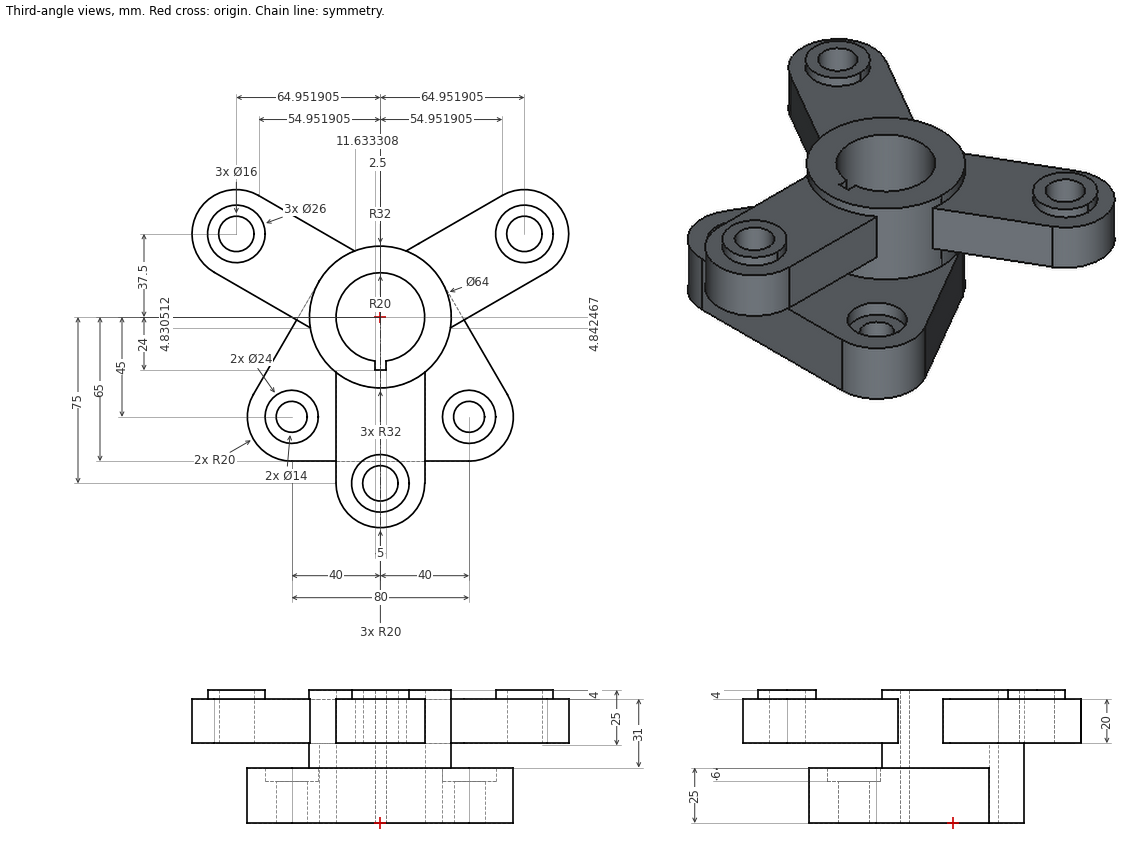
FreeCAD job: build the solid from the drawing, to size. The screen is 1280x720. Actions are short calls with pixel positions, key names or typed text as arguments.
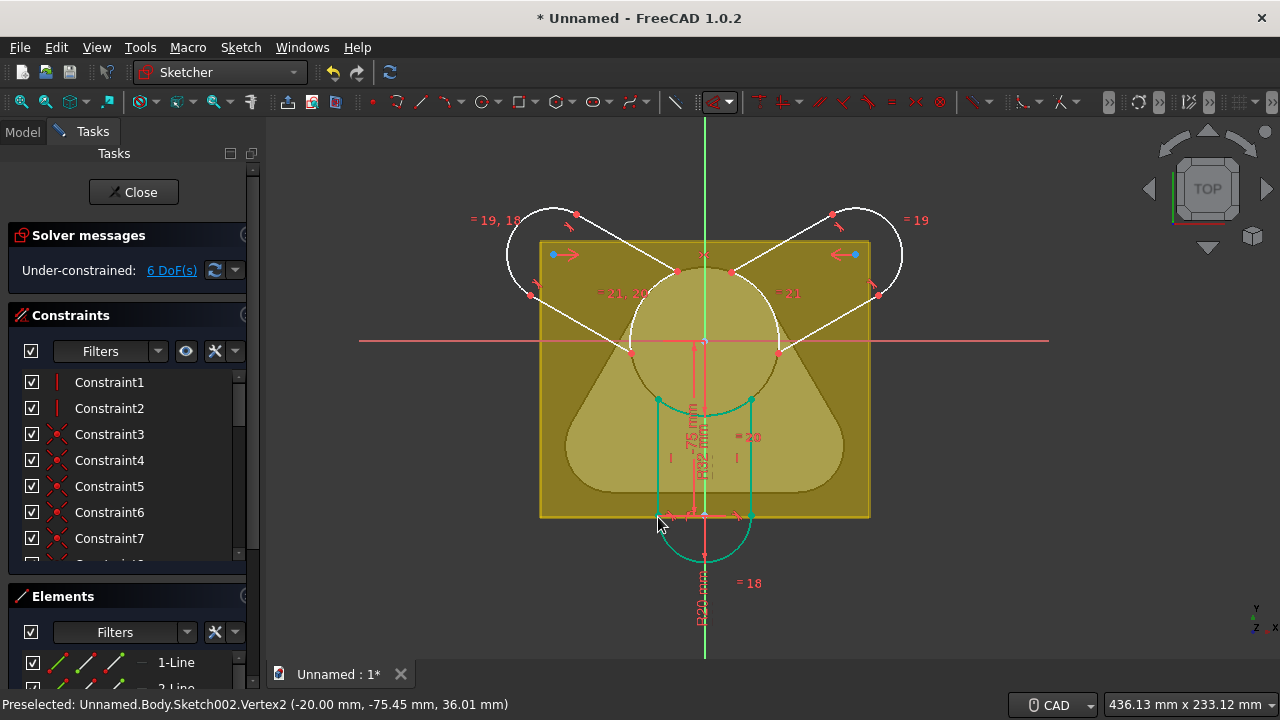
click(554, 255)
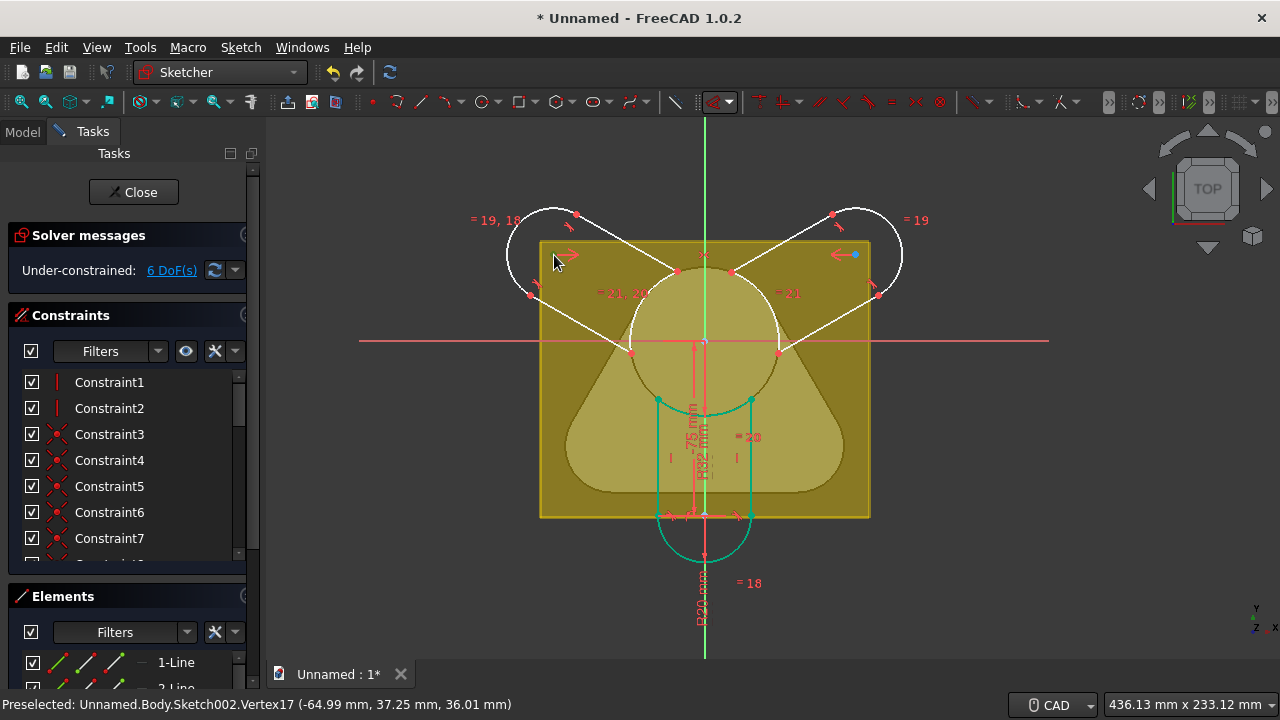
key(i)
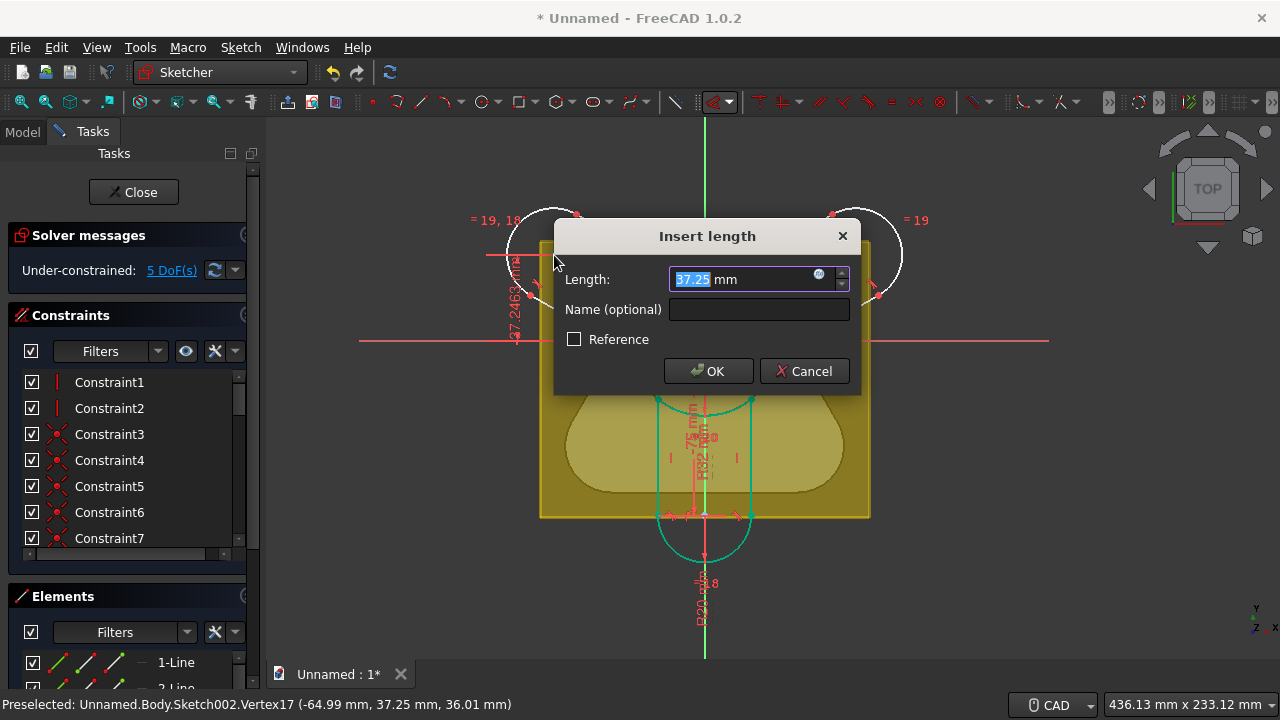
text(37.5)
key(Return)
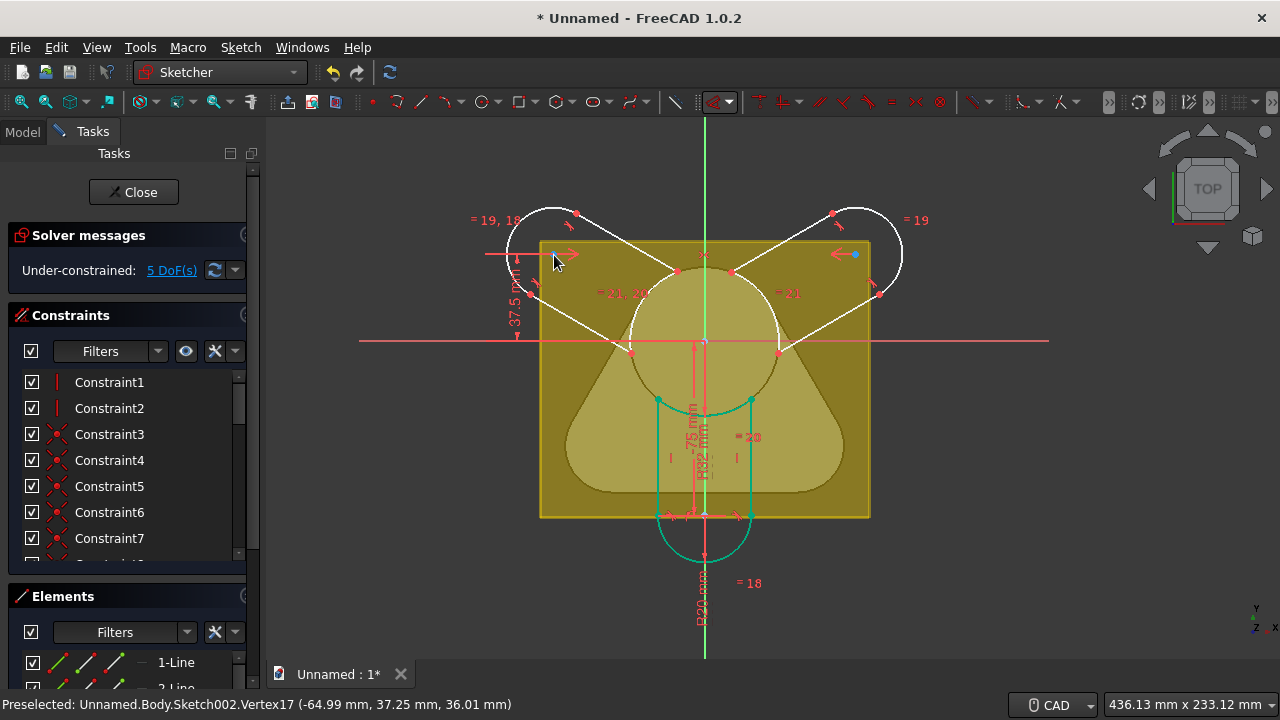
scroll(631, 353, up, 7)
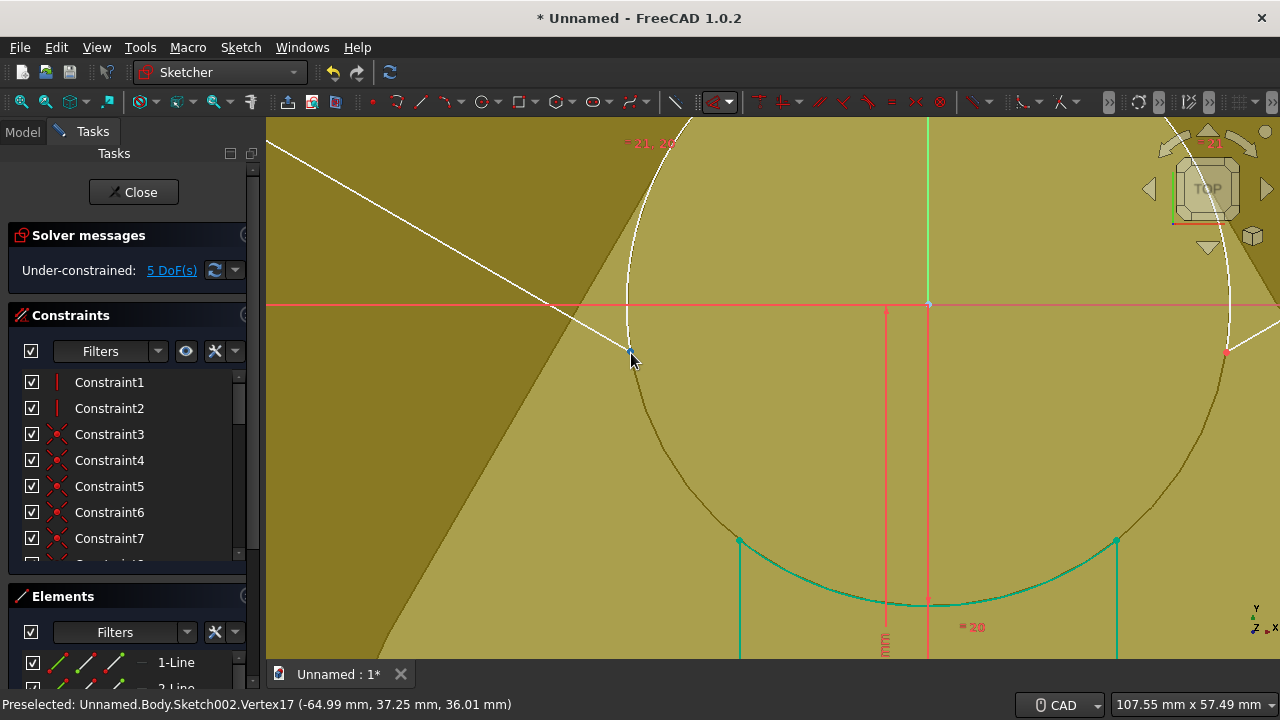
click(630, 352)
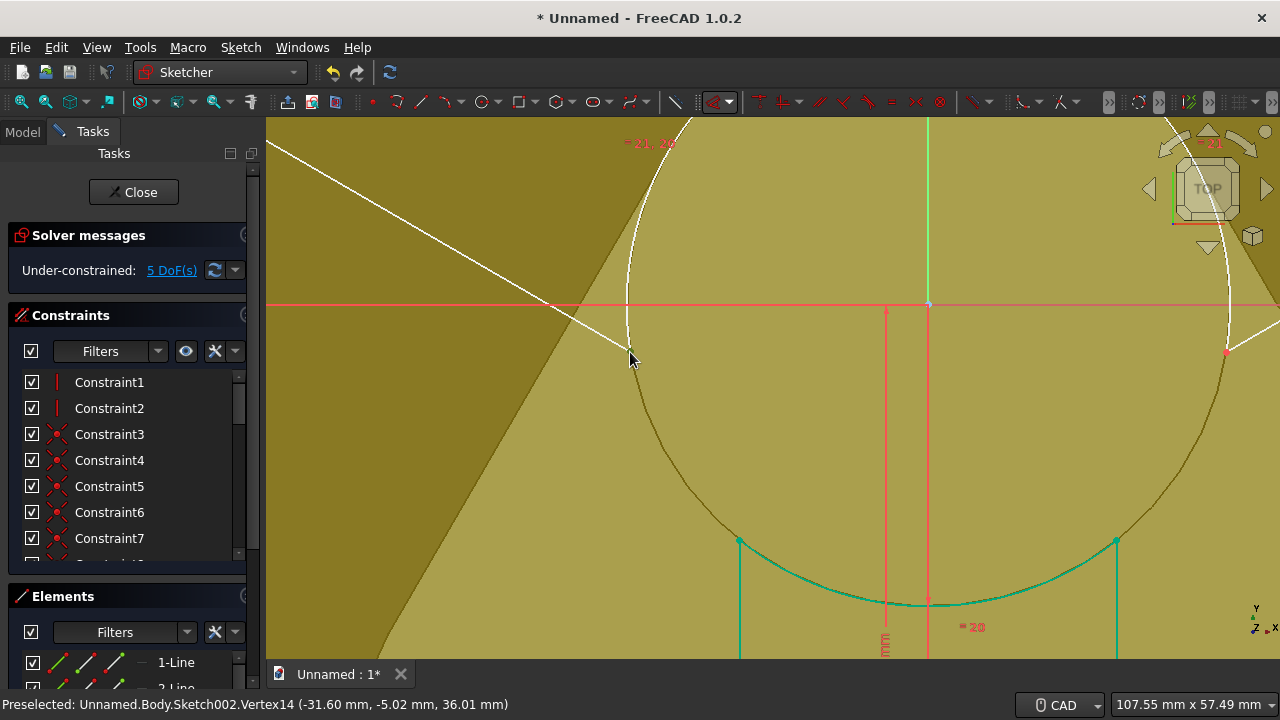
click(732, 102)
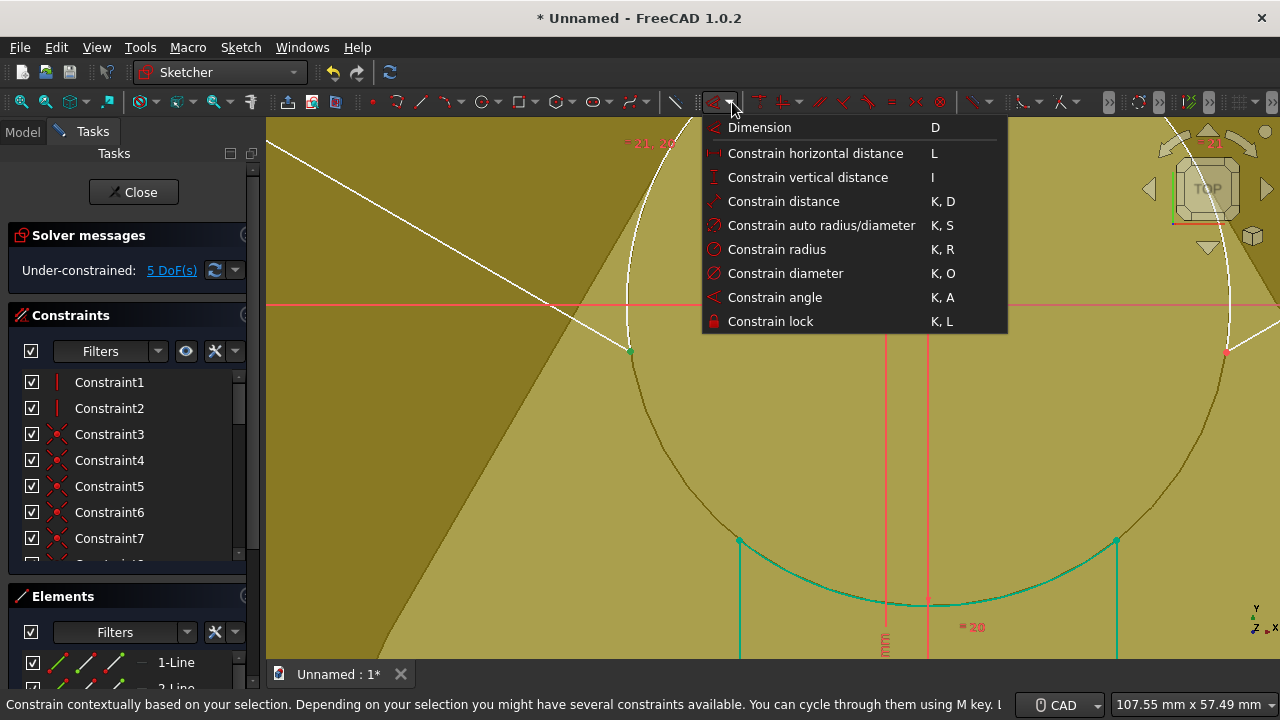
click(855, 177)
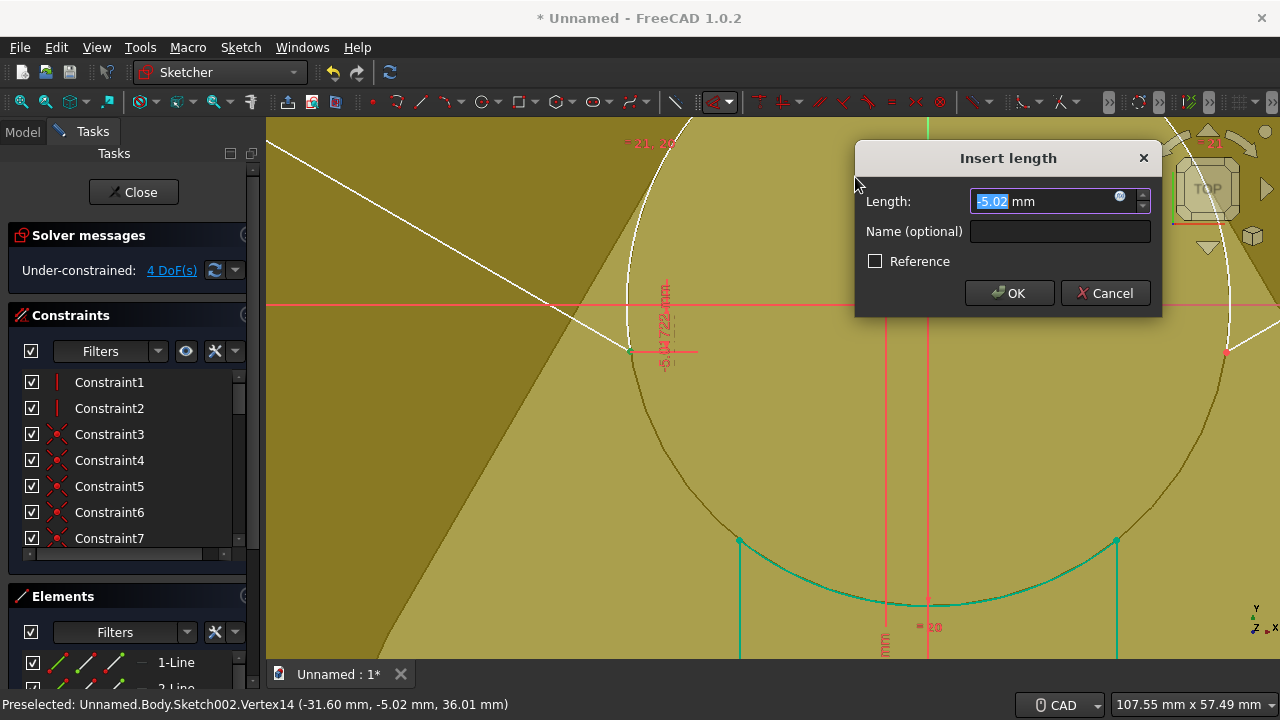
text(-4.830512)
key(Return)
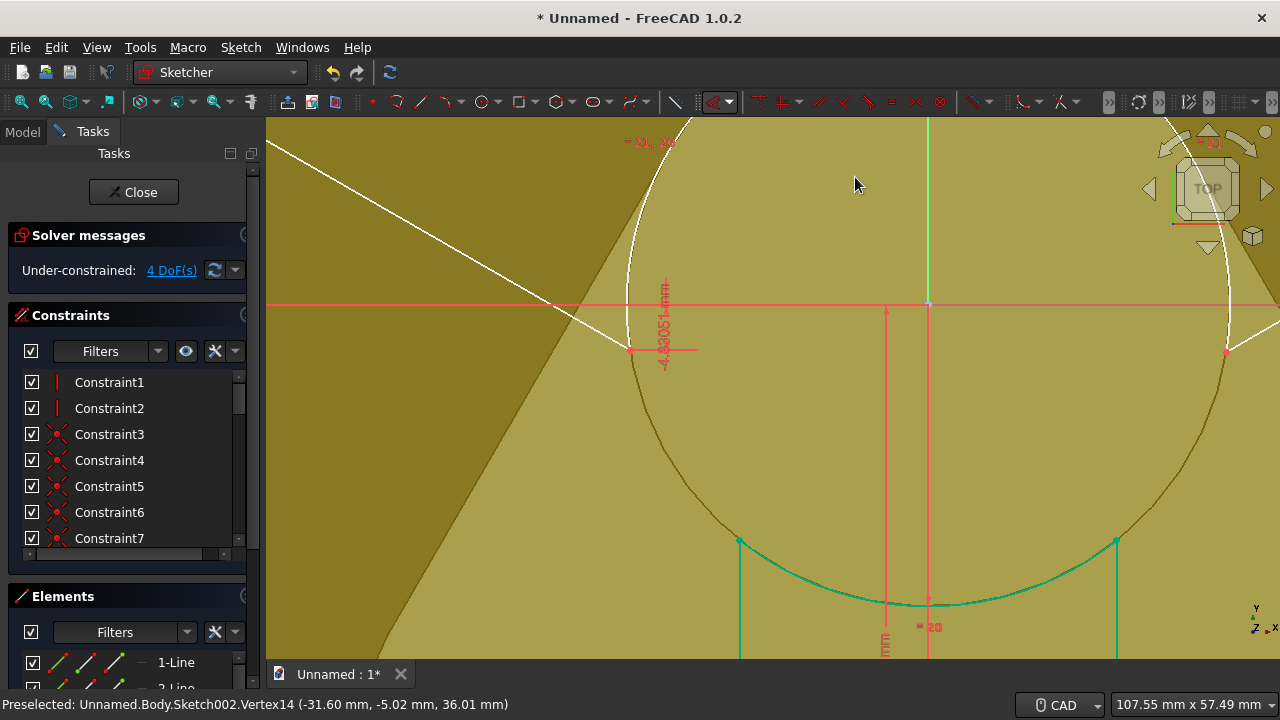
scroll(631, 353, down, 7)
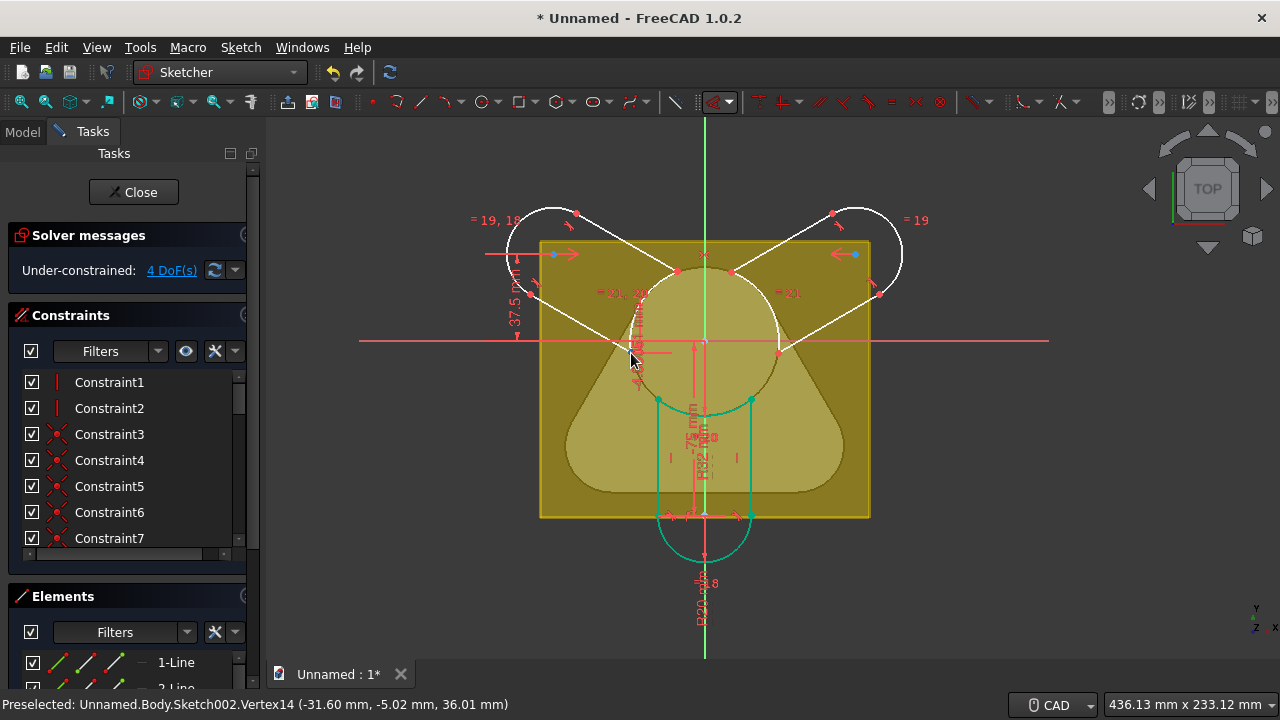
scroll(778, 353, up, 7)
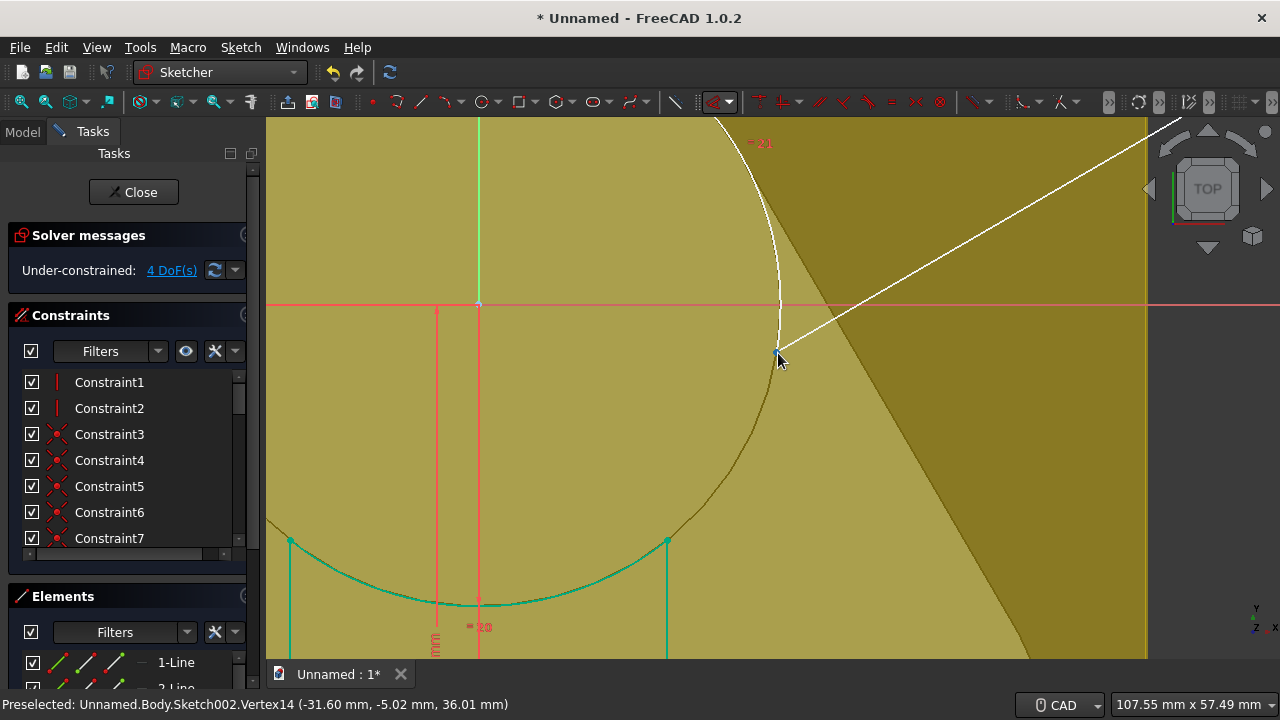
click(777, 352)